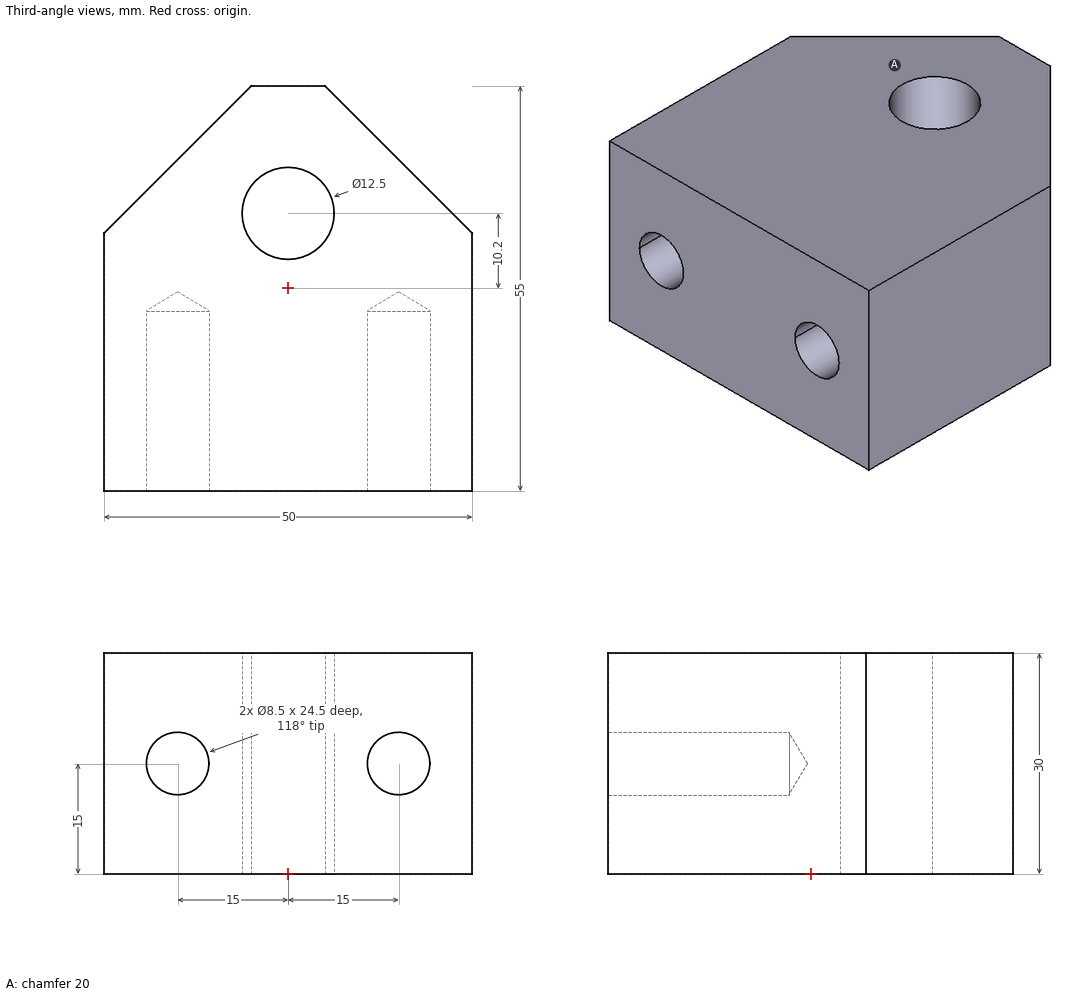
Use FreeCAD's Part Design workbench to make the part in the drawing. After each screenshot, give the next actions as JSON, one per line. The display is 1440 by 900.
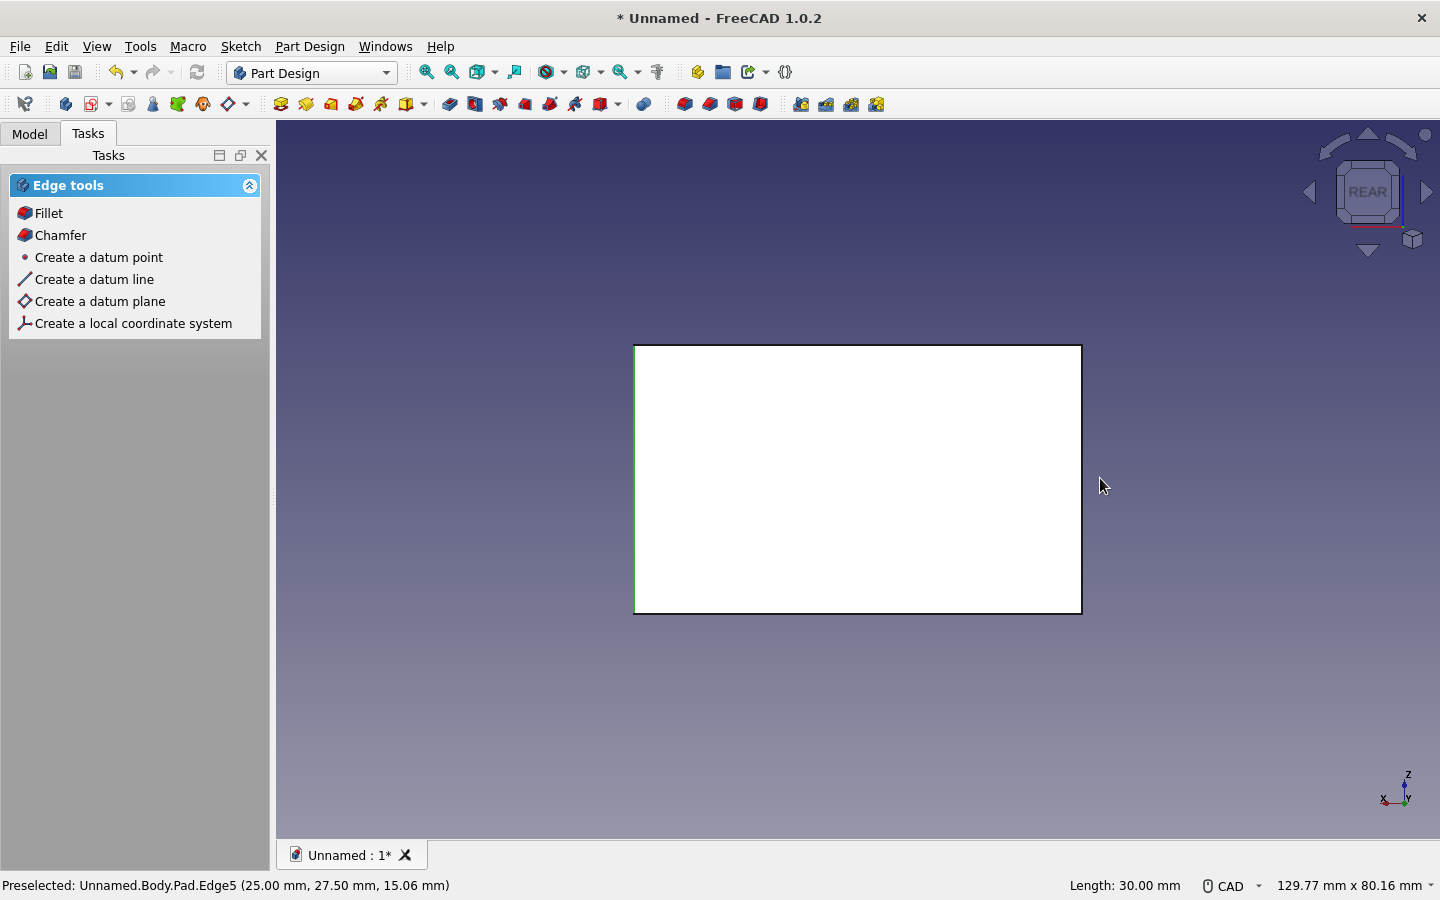
{"action": "left_click", "coordinate": [427, 72]}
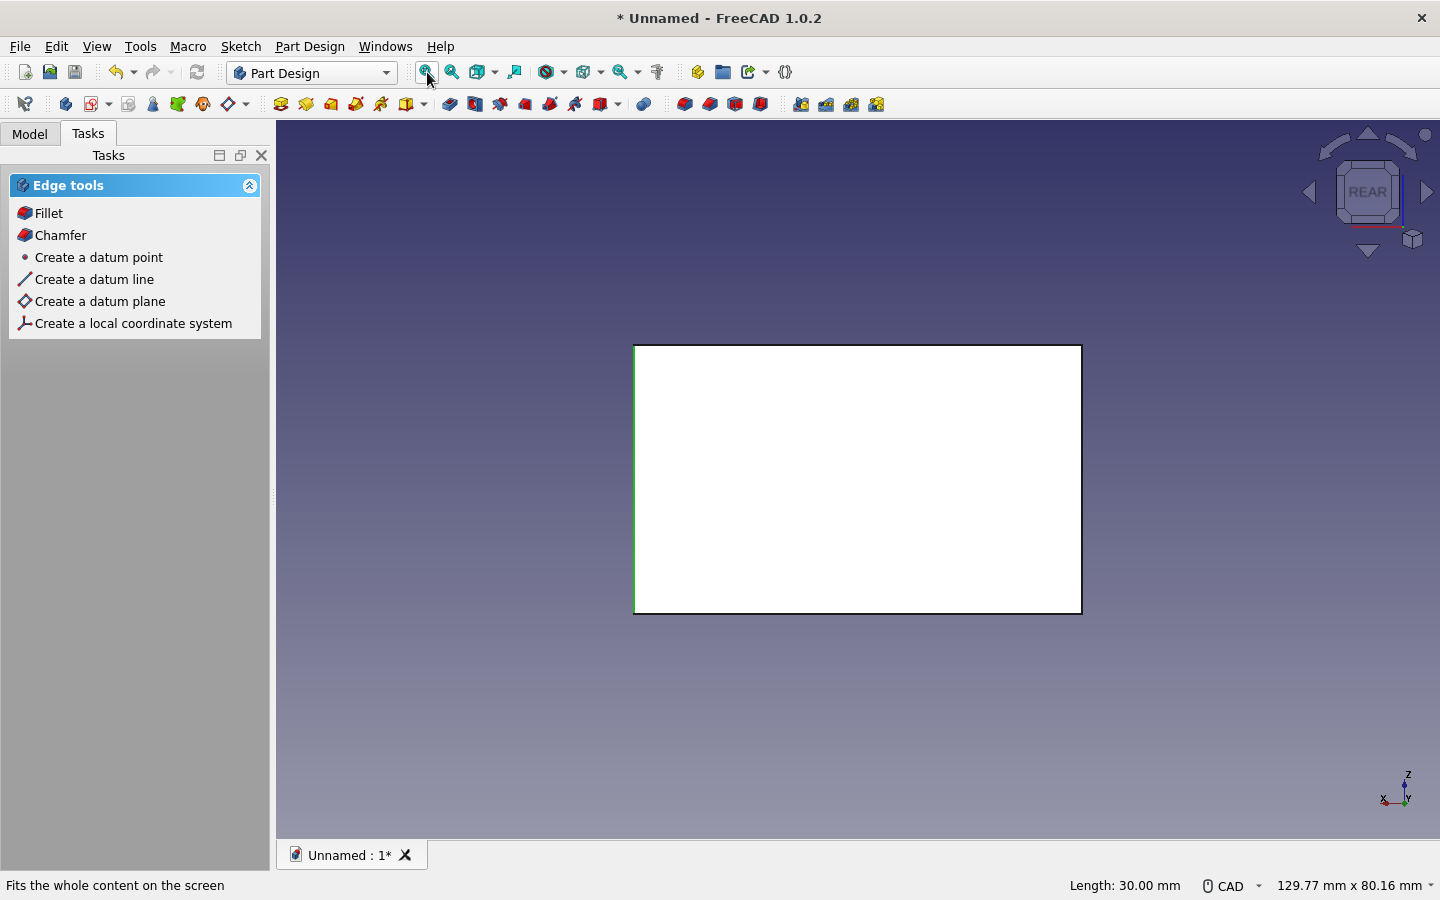
{"action": "left_click", "coordinate": [1082, 479], "text": "ctrl"}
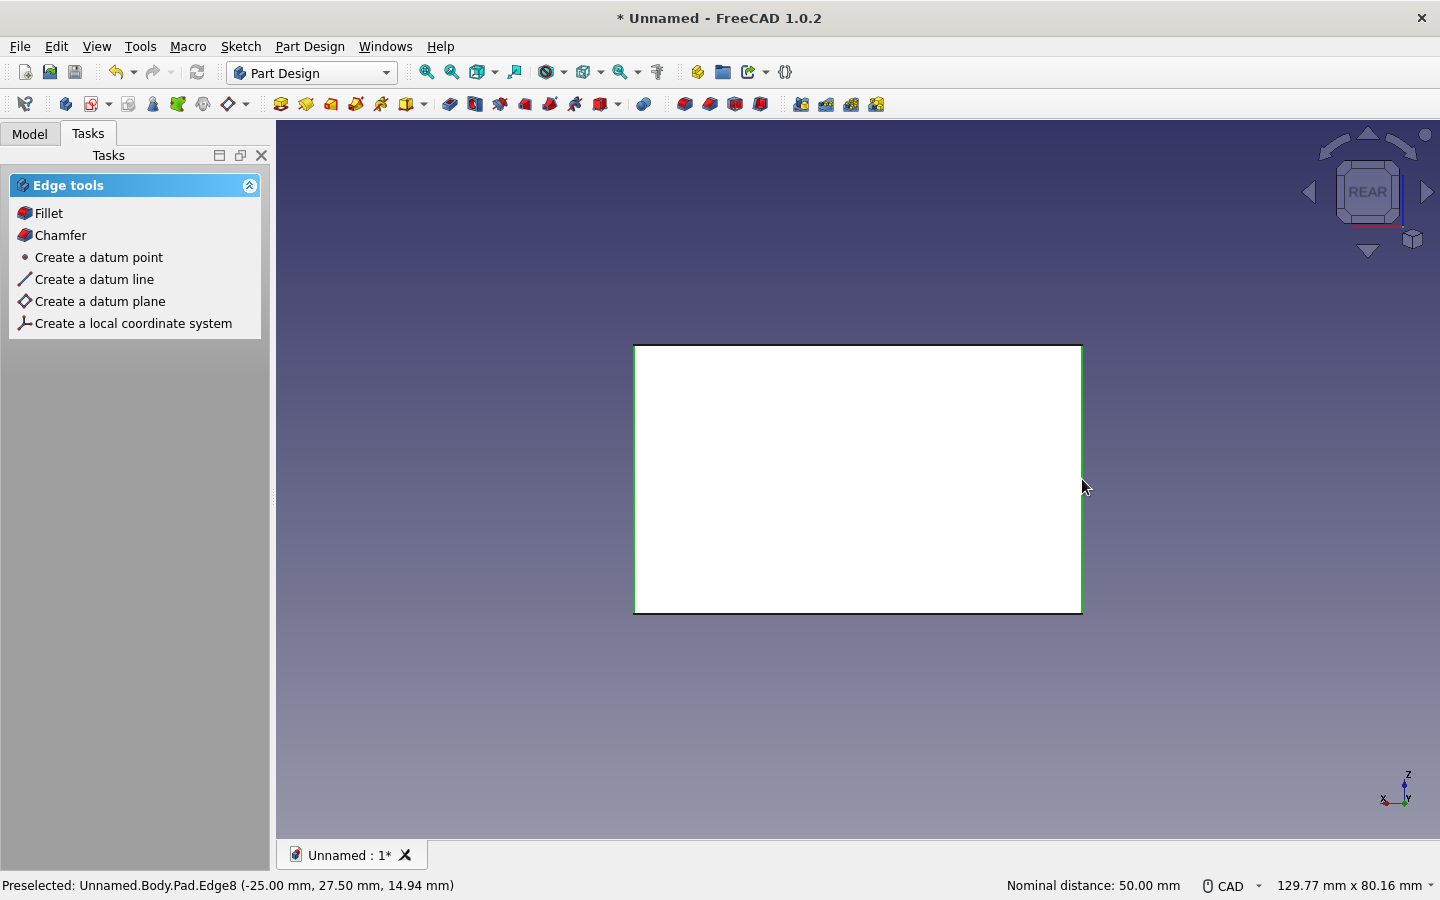
{"action": "left_click", "coordinate": [710, 104]}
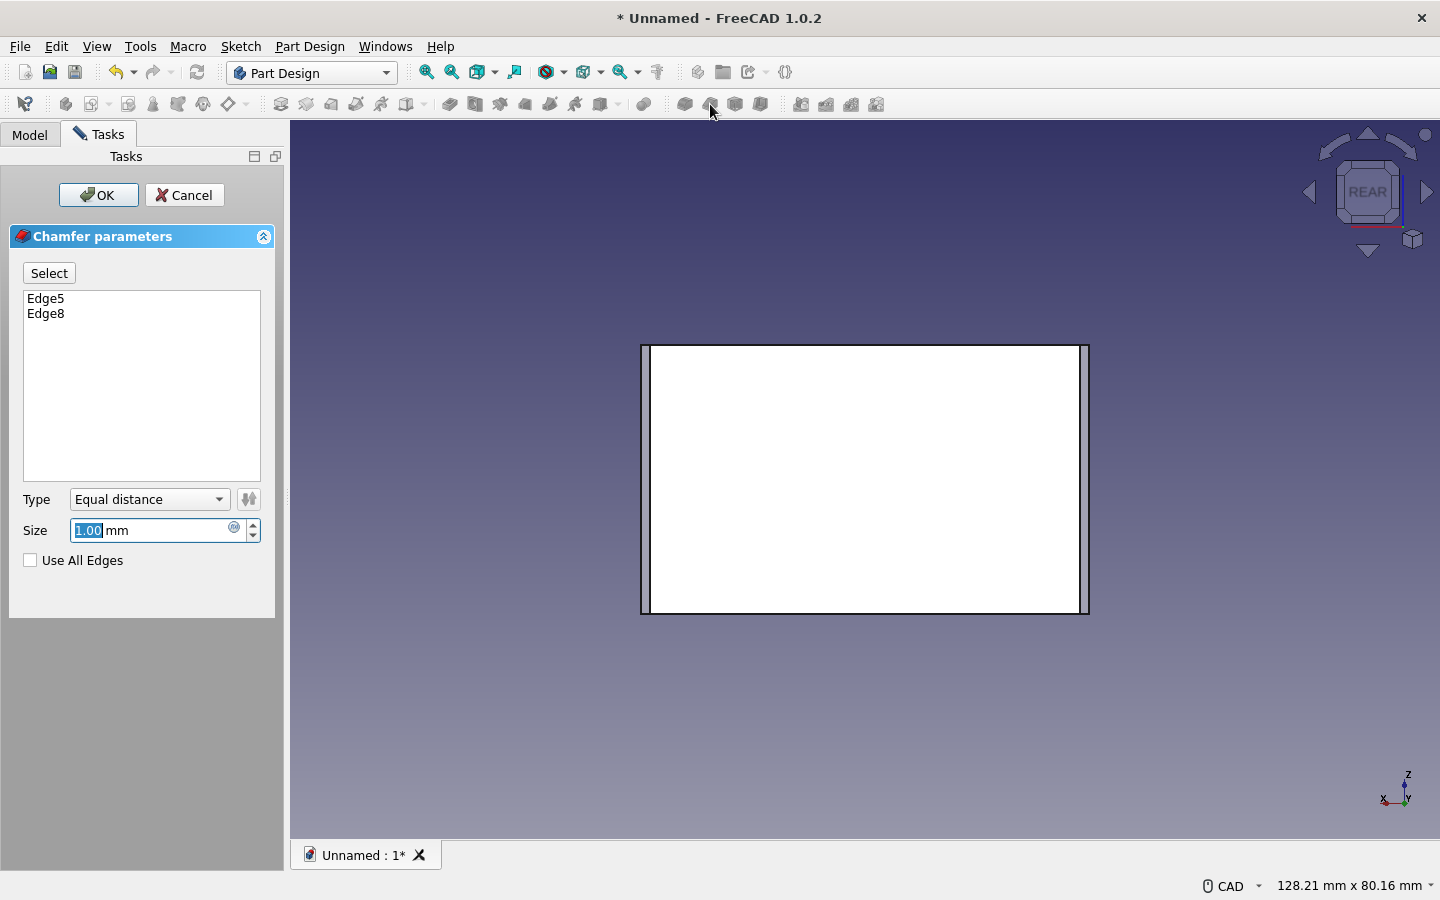
{"action": "type", "text": "20"}
{"action": "key", "text": "Tab"}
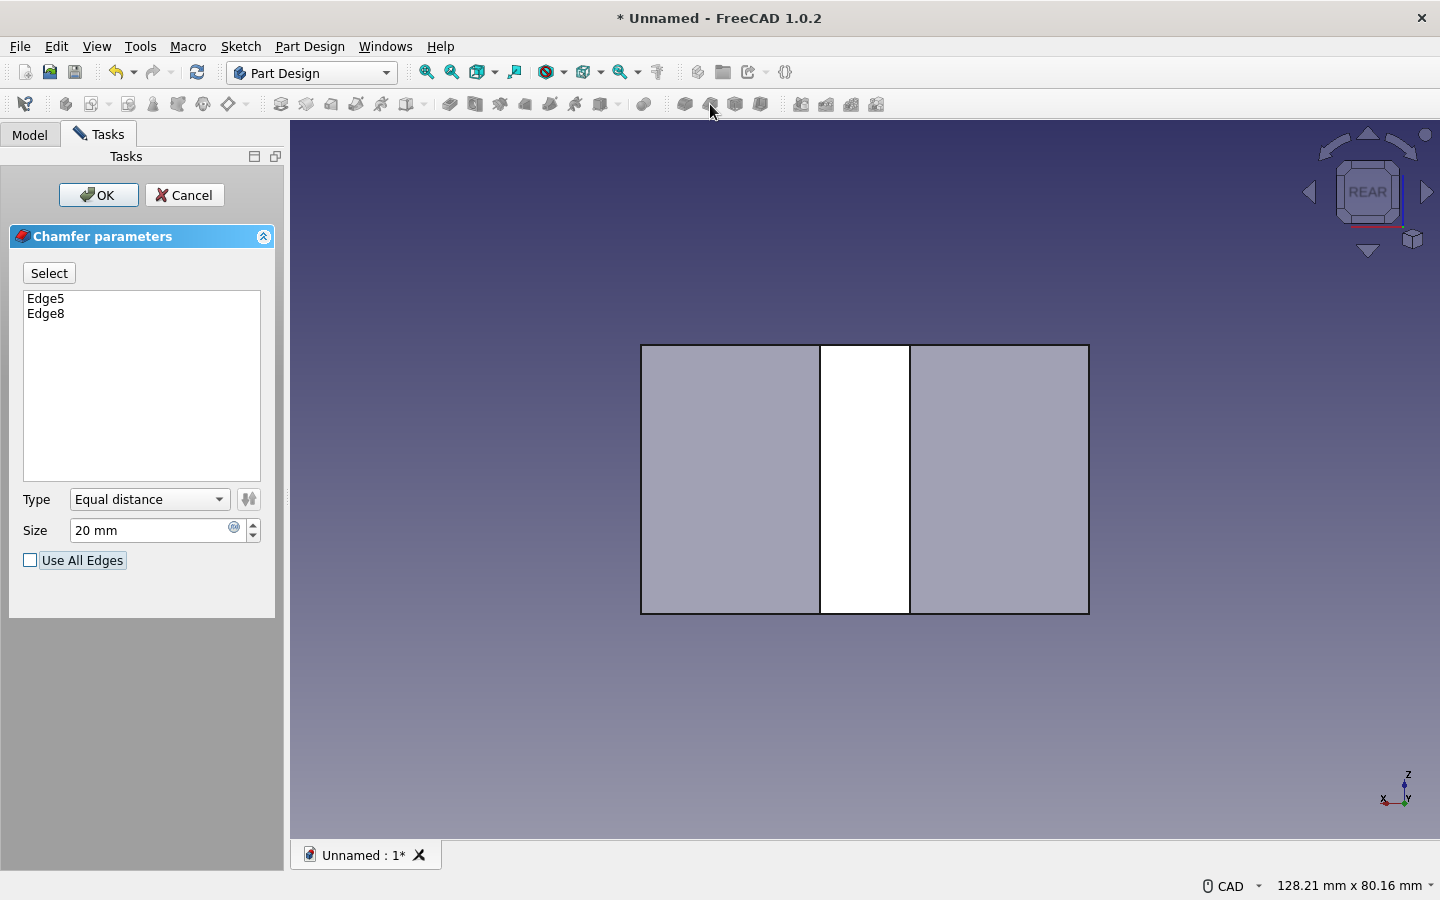
{"action": "left_click", "coordinate": [99, 195]}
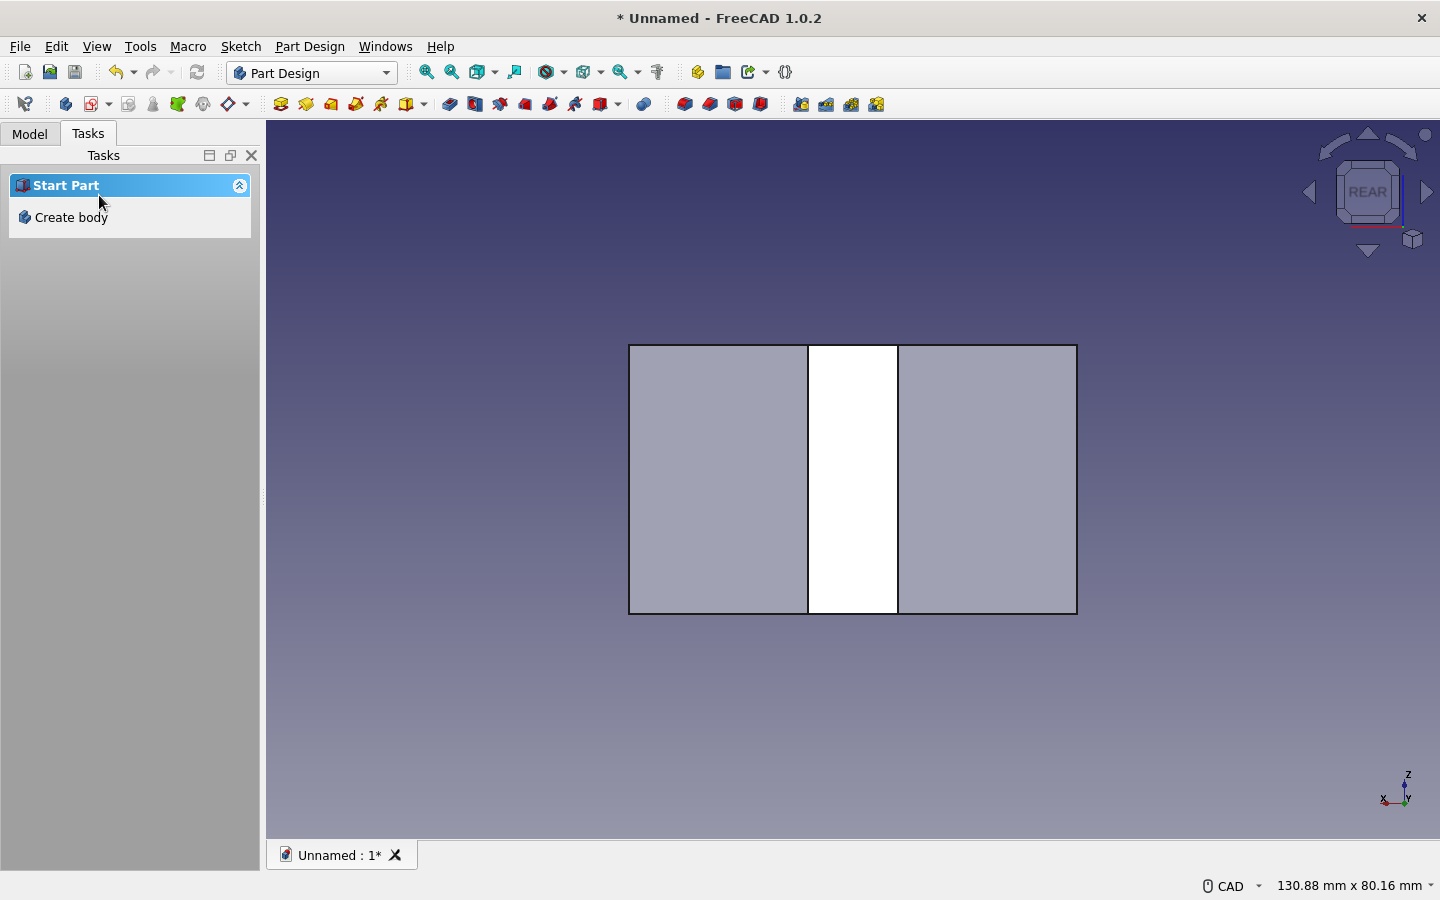
{"action": "key", "text": "v f"}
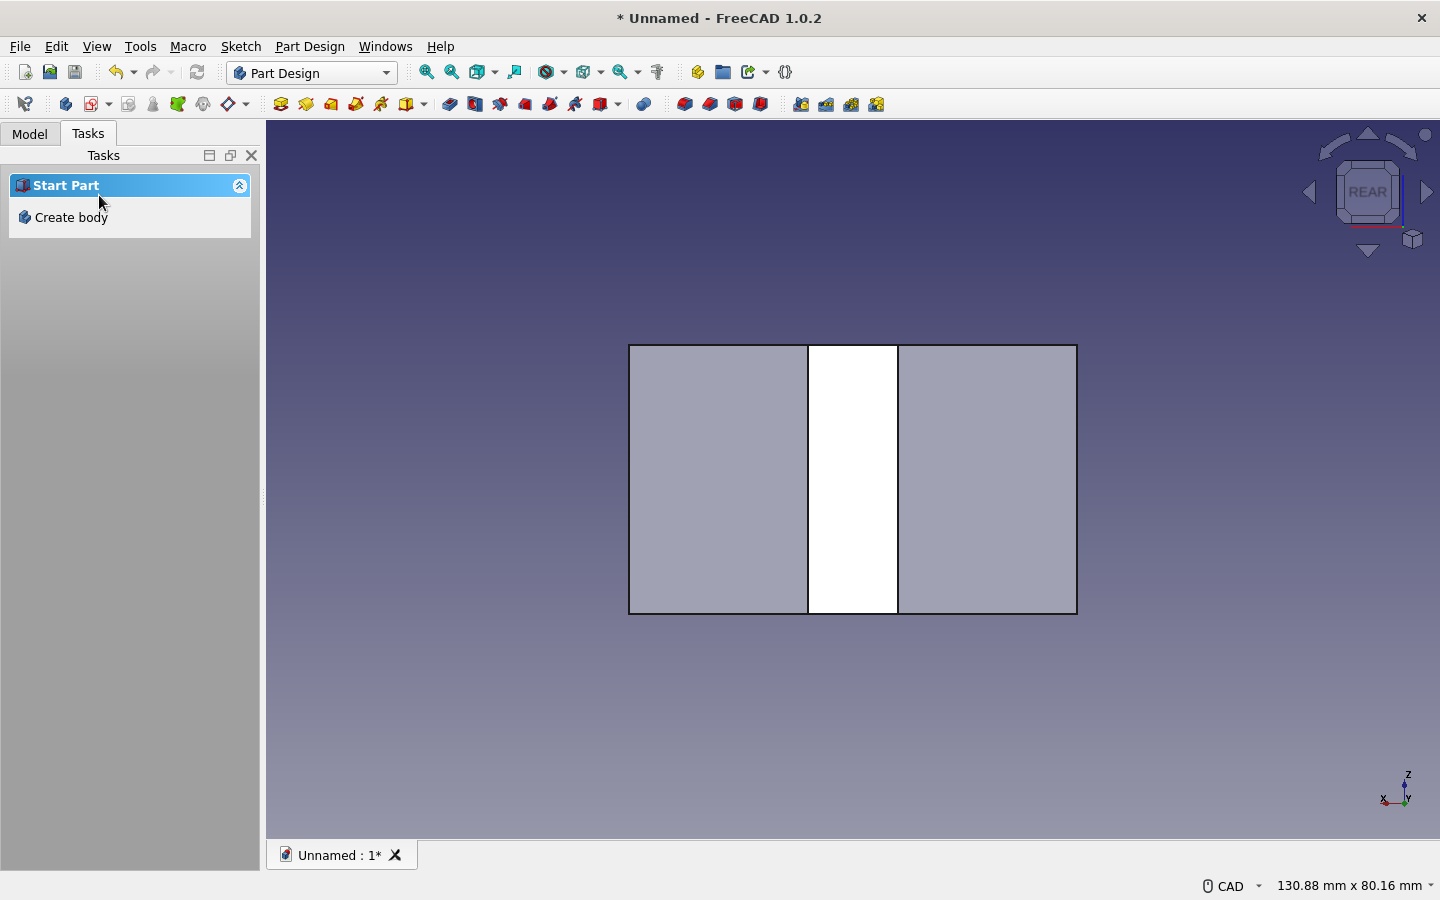
{"action": "key", "text": "0"}